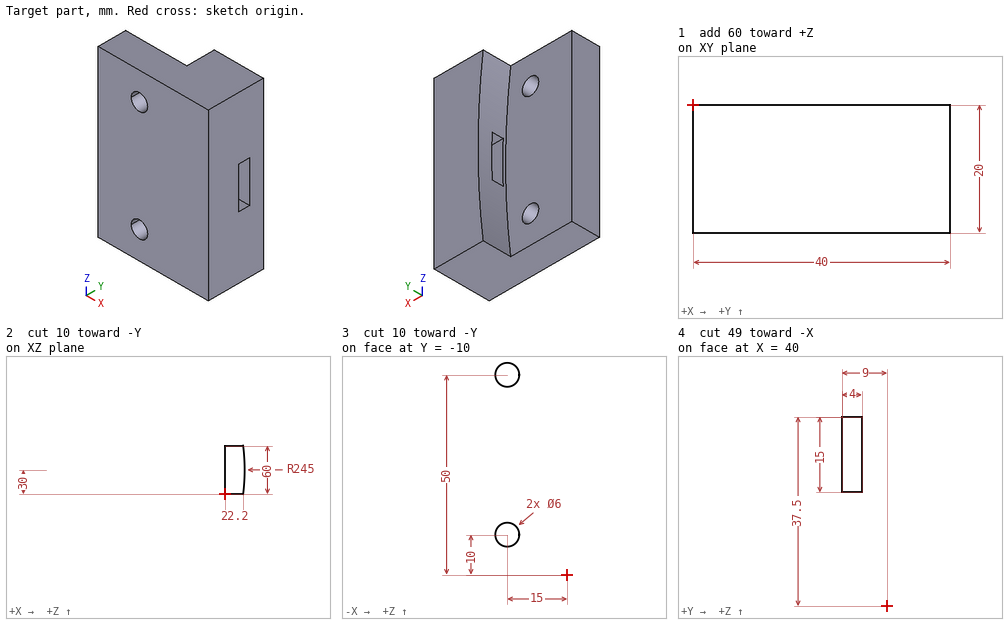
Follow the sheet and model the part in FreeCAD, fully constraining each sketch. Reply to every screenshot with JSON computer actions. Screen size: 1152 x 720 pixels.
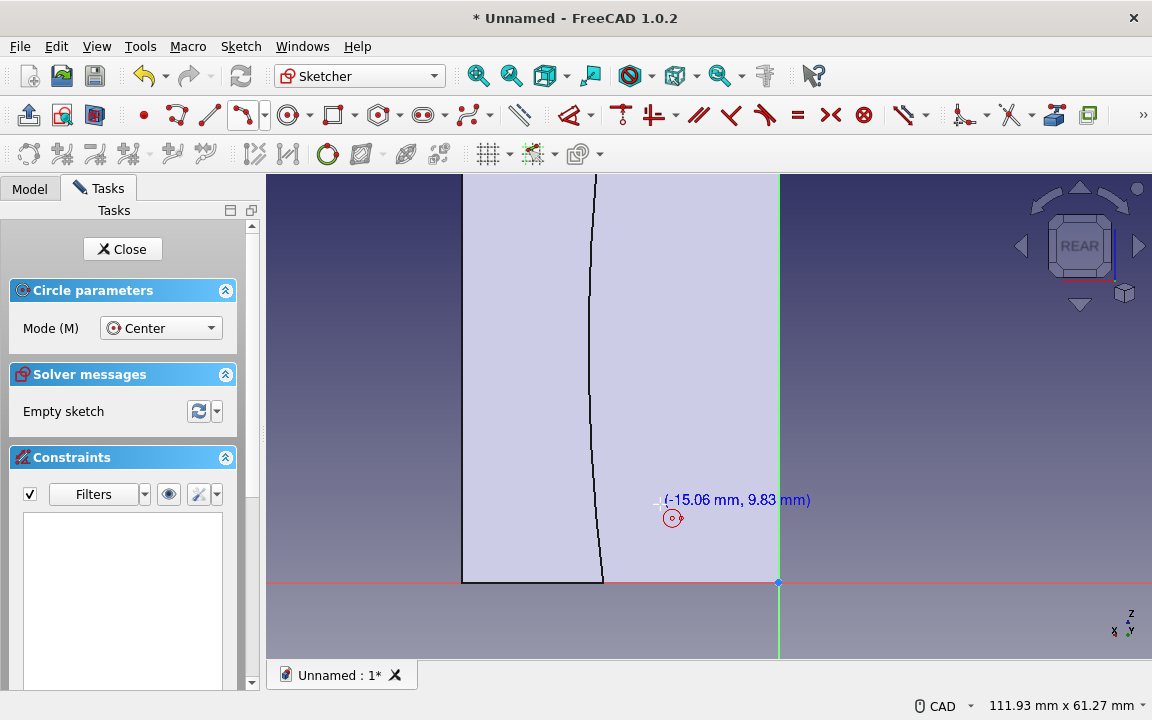
{"action": "left_click", "coordinate": [660, 504]}
{"action": "mouse_move", "coordinate": [677, 487]}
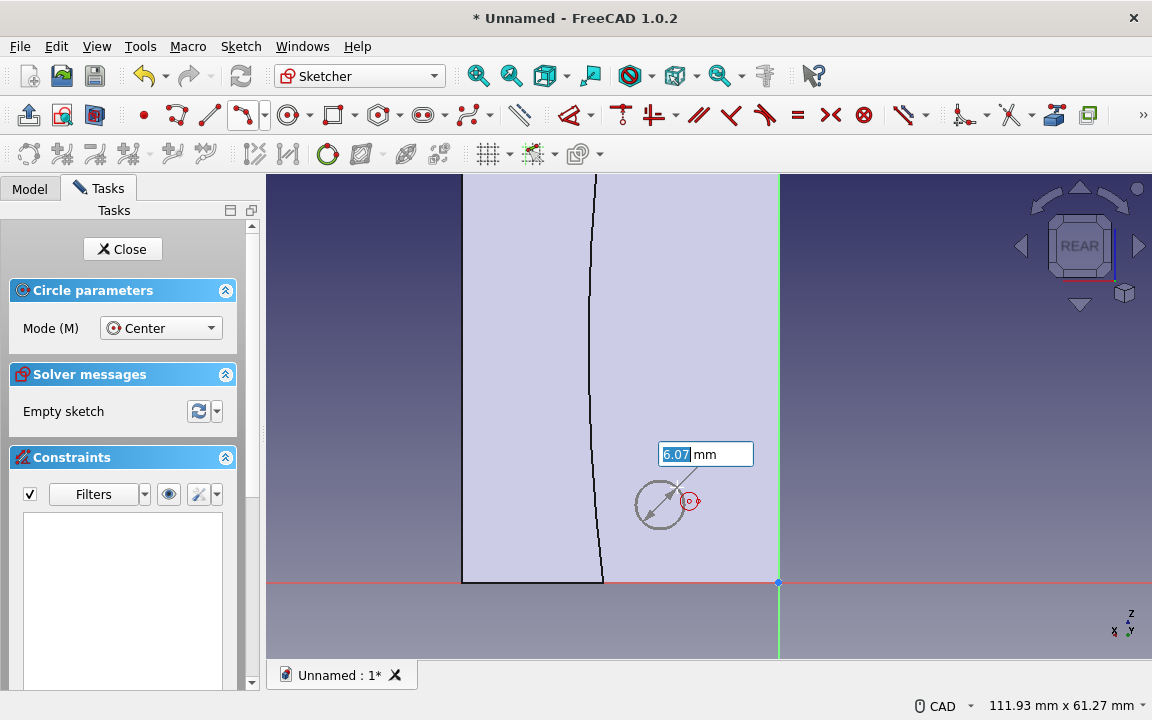
{"action": "type", "text": "6"}
{"action": "key", "text": "Return"}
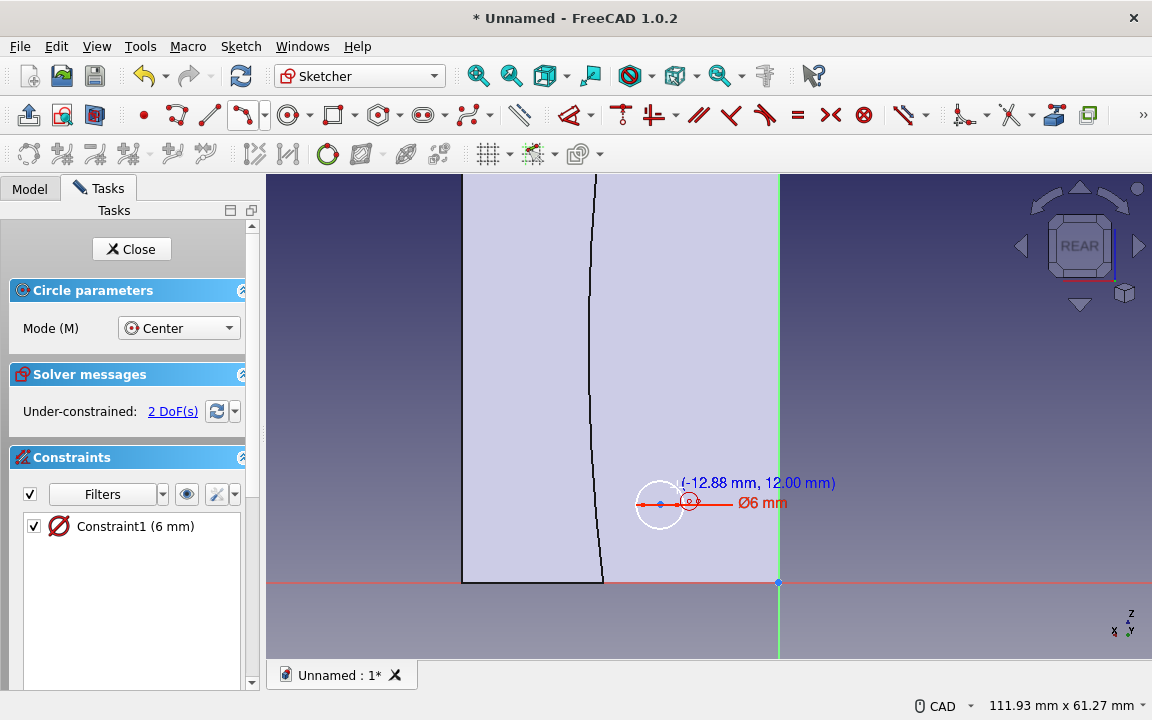
{"action": "scroll", "coordinate": [504, 505], "scroll_direction": "down", "scroll_amount": 2}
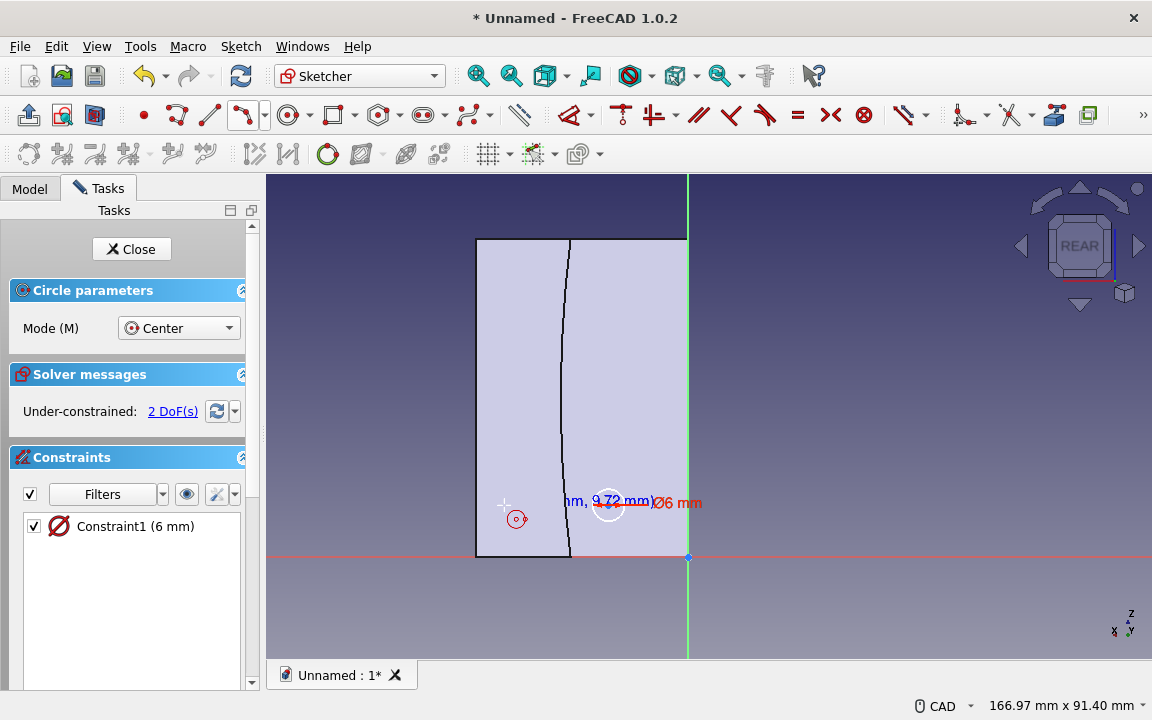
{"action": "scroll", "coordinate": [609, 292], "scroll_direction": "up", "scroll_amount": 2}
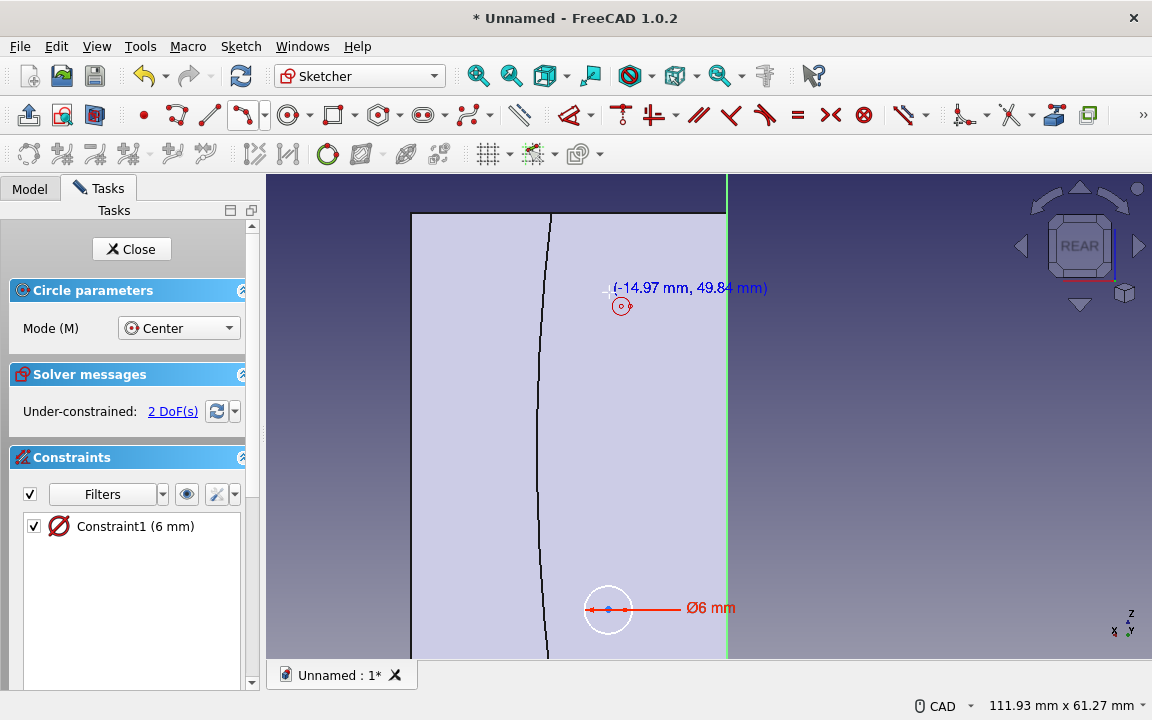
{"action": "left_click", "coordinate": [609, 292]}
{"action": "mouse_move", "coordinate": [625, 275]}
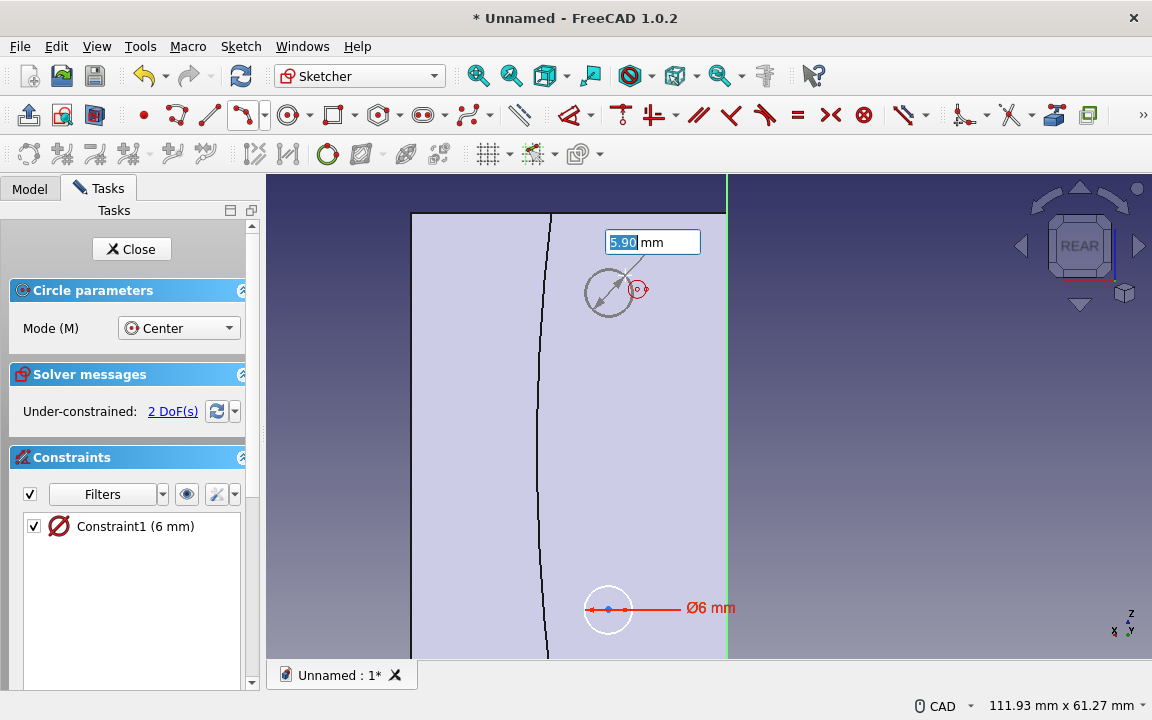
{"action": "type", "text": "6"}
{"action": "key", "text": "Return"}
{"action": "key", "text": "Escape"}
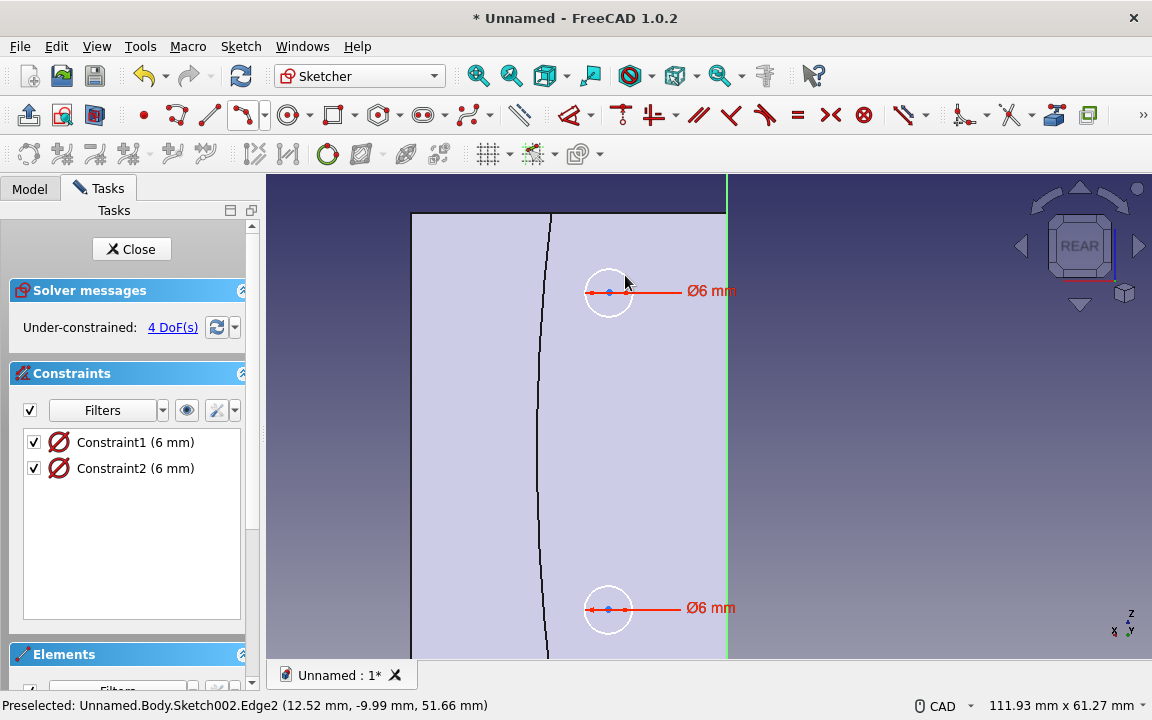
{"action": "left_click", "coordinate": [608, 610]}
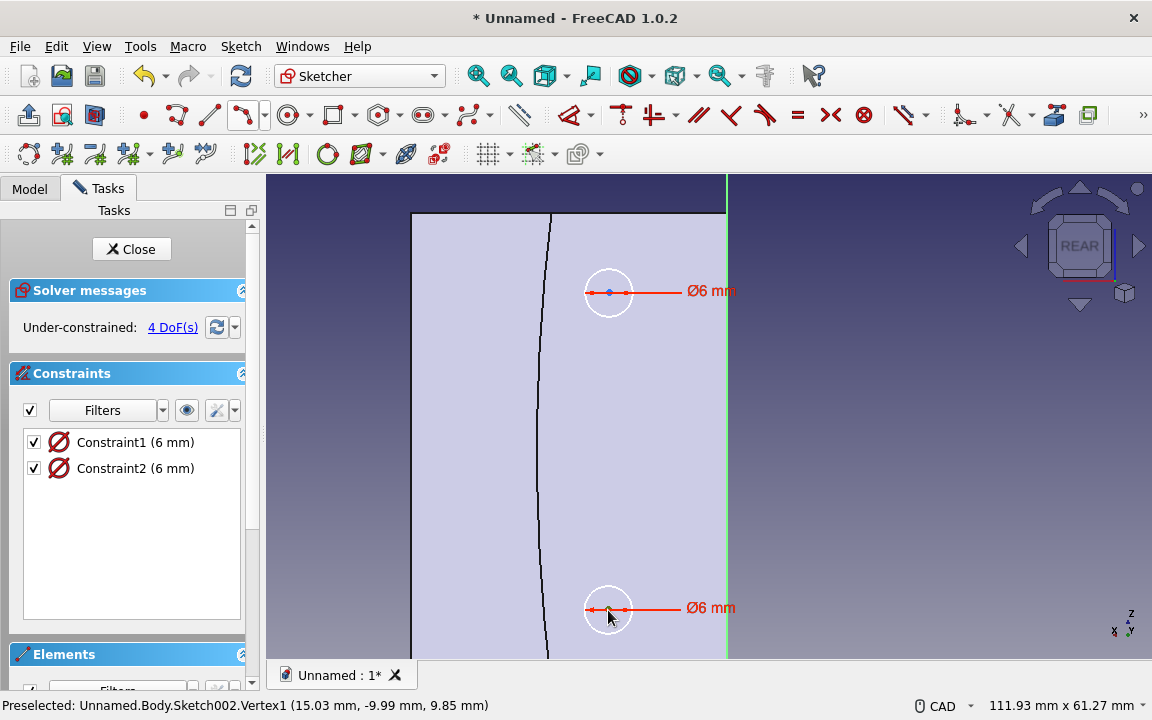
{"action": "left_click", "coordinate": [609, 293]}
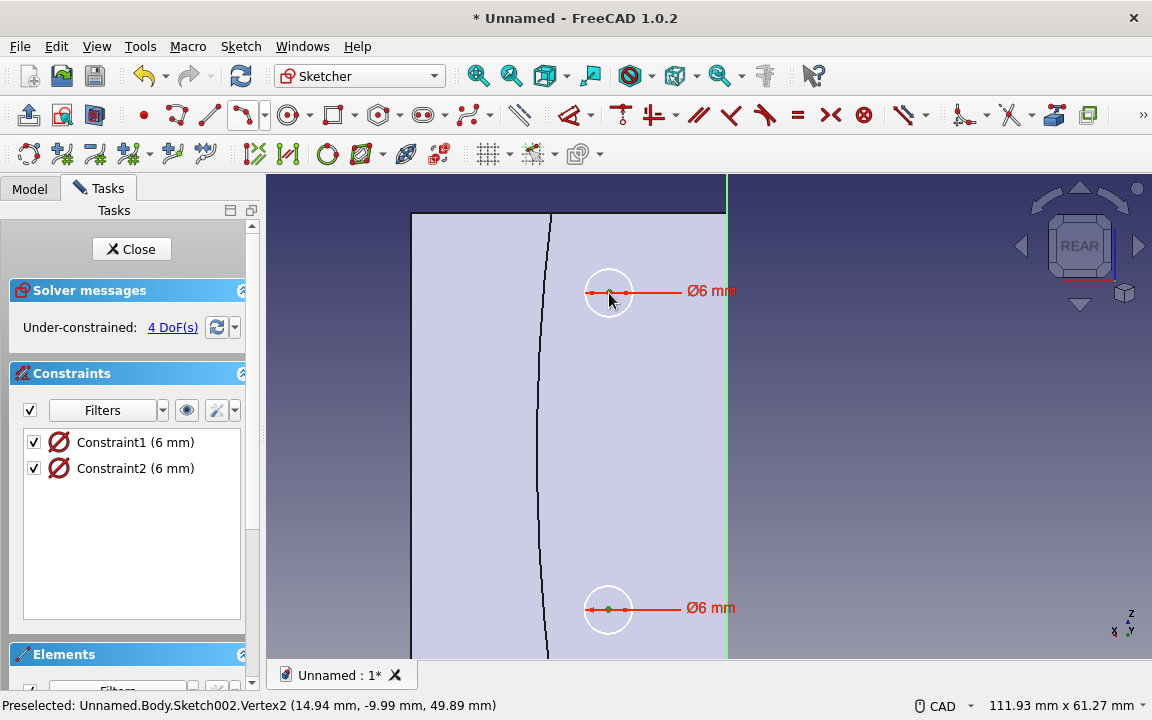
{"action": "key", "text": "v"}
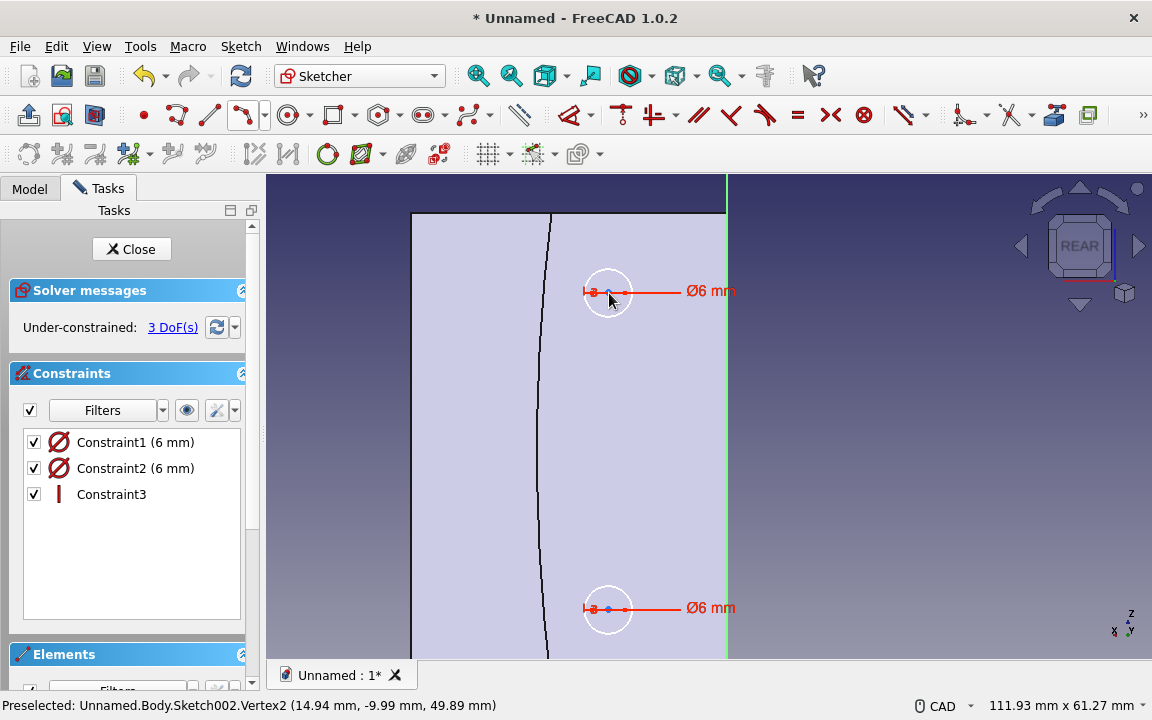
{"action": "left_click", "coordinate": [568, 116]}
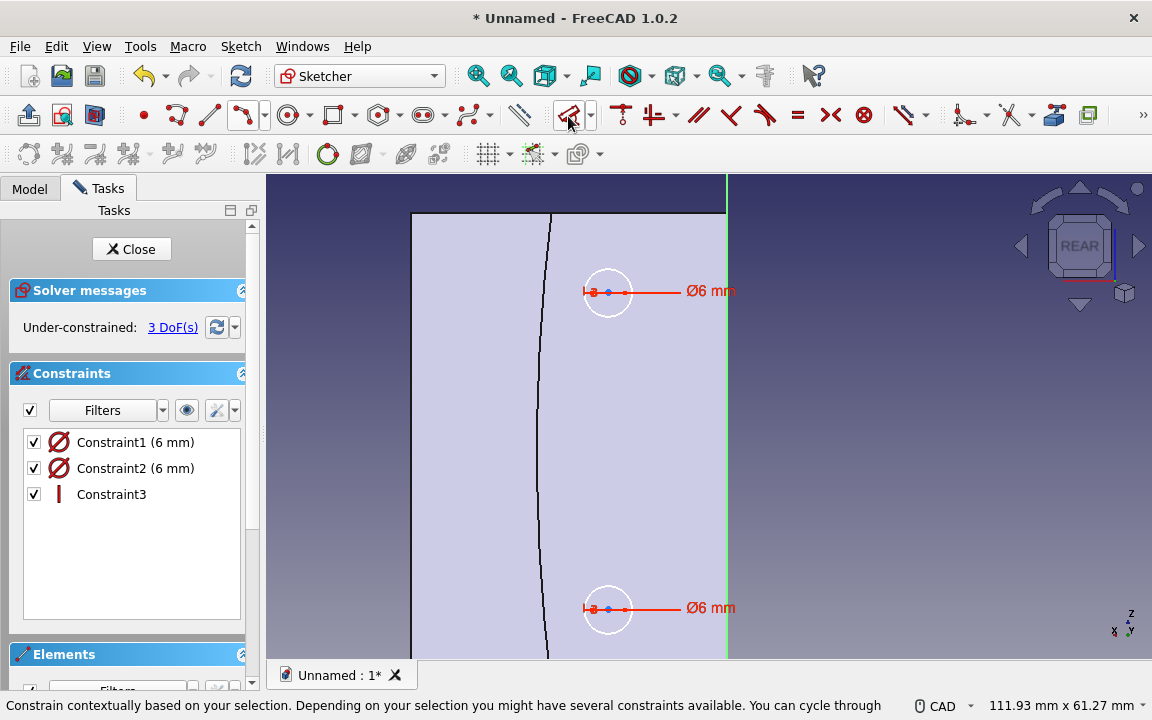
{"action": "left_click", "coordinate": [608, 610]}
{"action": "left_click", "coordinate": [668, 576]}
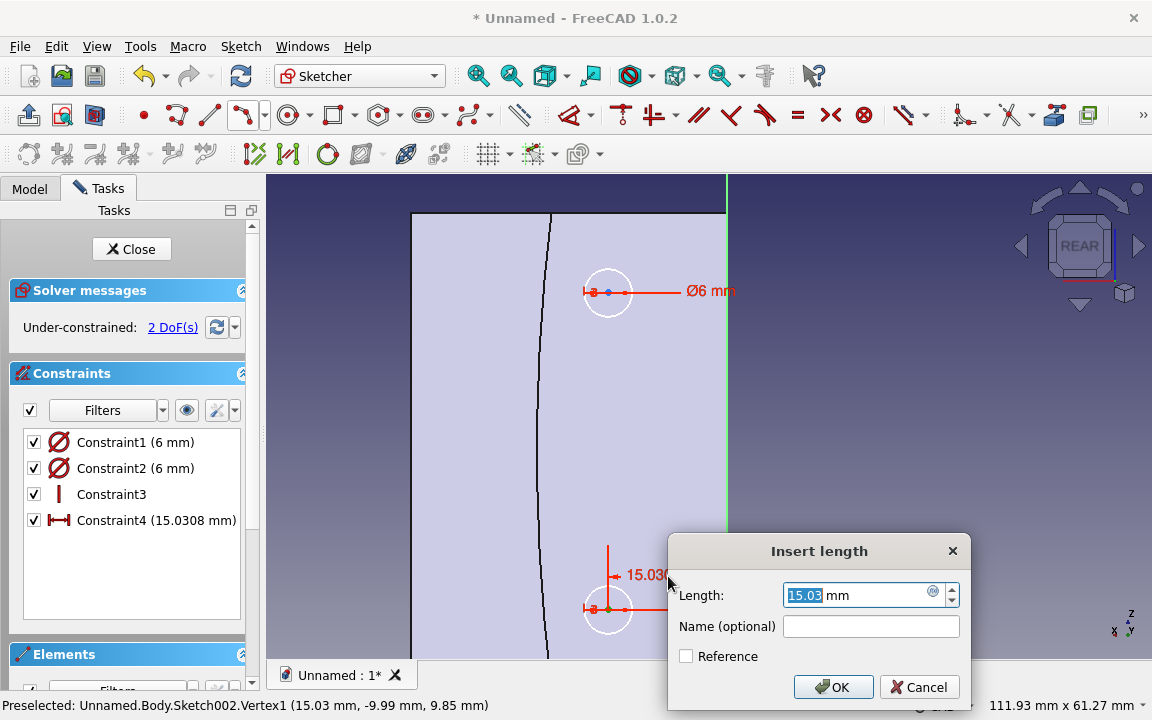
{"action": "type", "text": "15"}
{"action": "key", "text": "Return"}